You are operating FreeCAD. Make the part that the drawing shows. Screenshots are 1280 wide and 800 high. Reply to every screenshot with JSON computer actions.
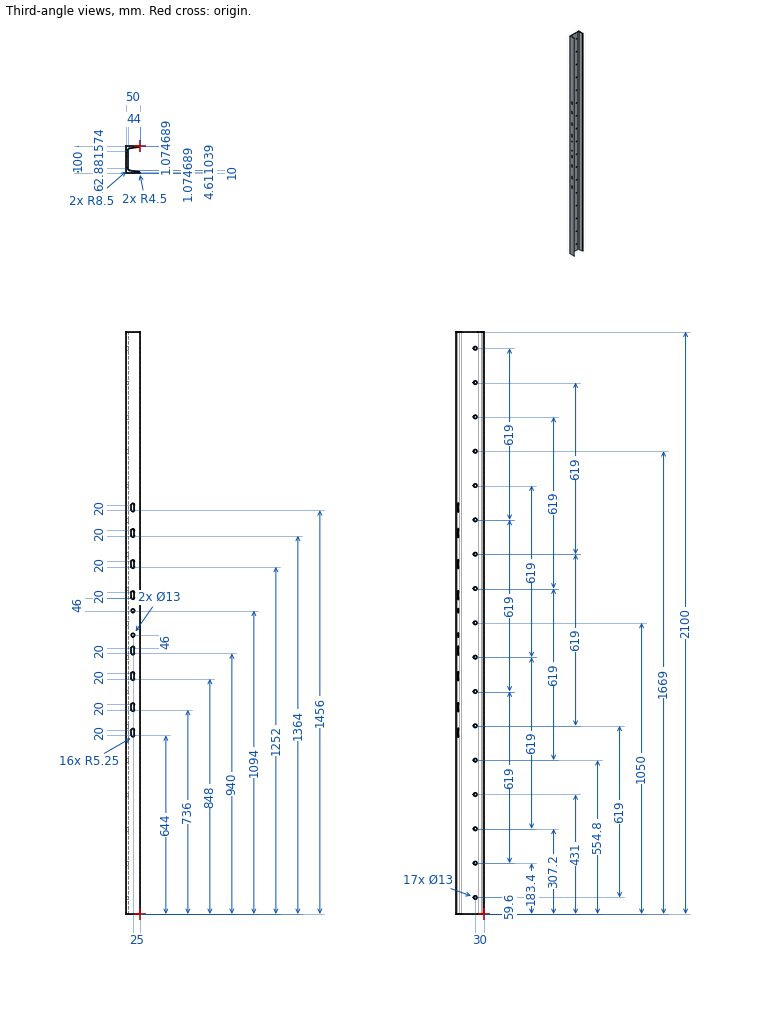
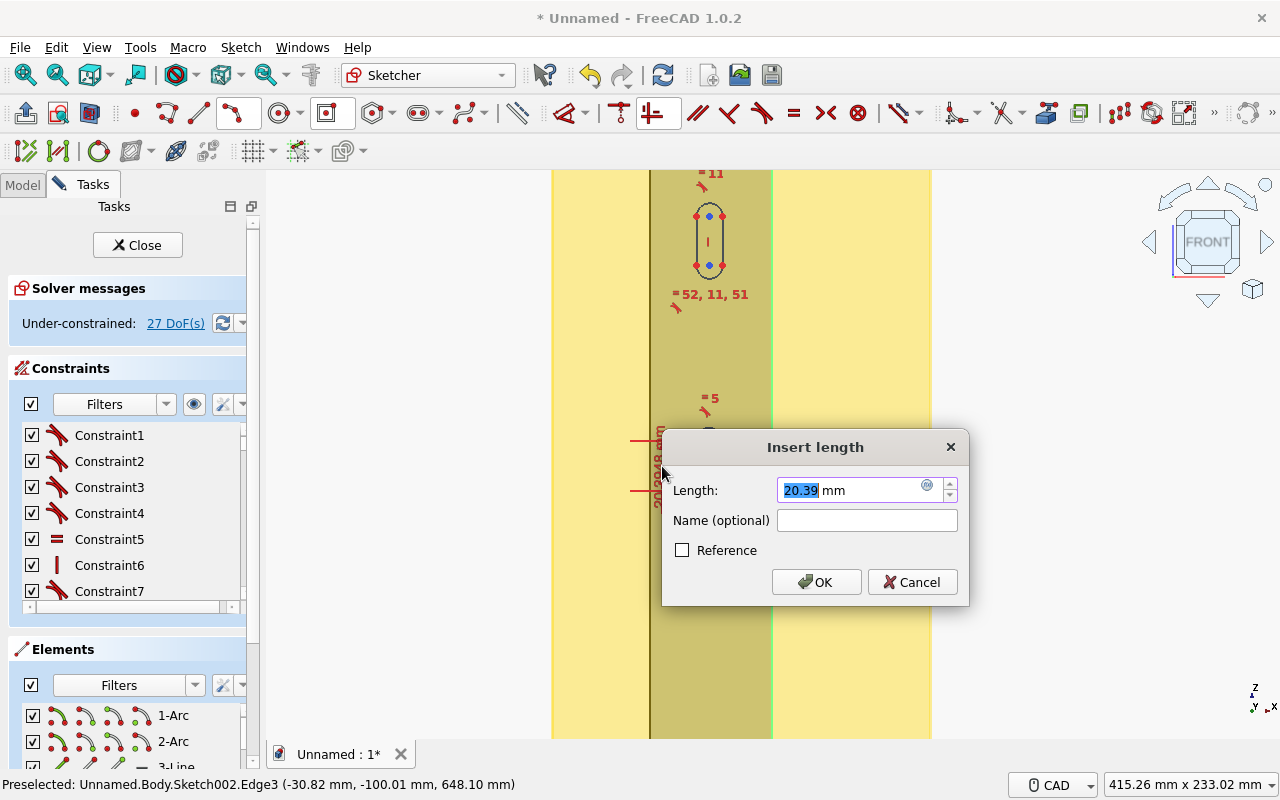
{"action": "type", "text": "20"}
{"action": "key", "text": "Return"}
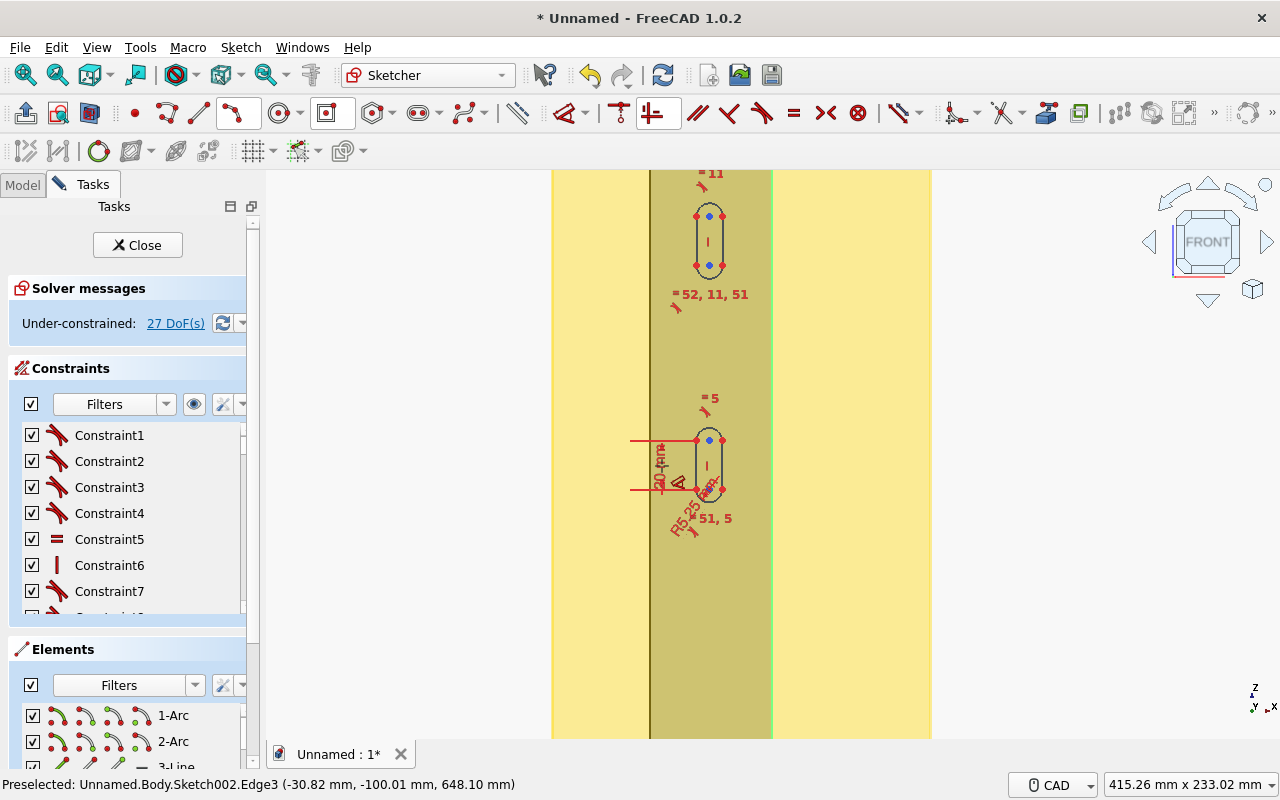
{"action": "left_click", "coordinate": [697, 251]}
{"action": "left_click", "coordinate": [663, 241]}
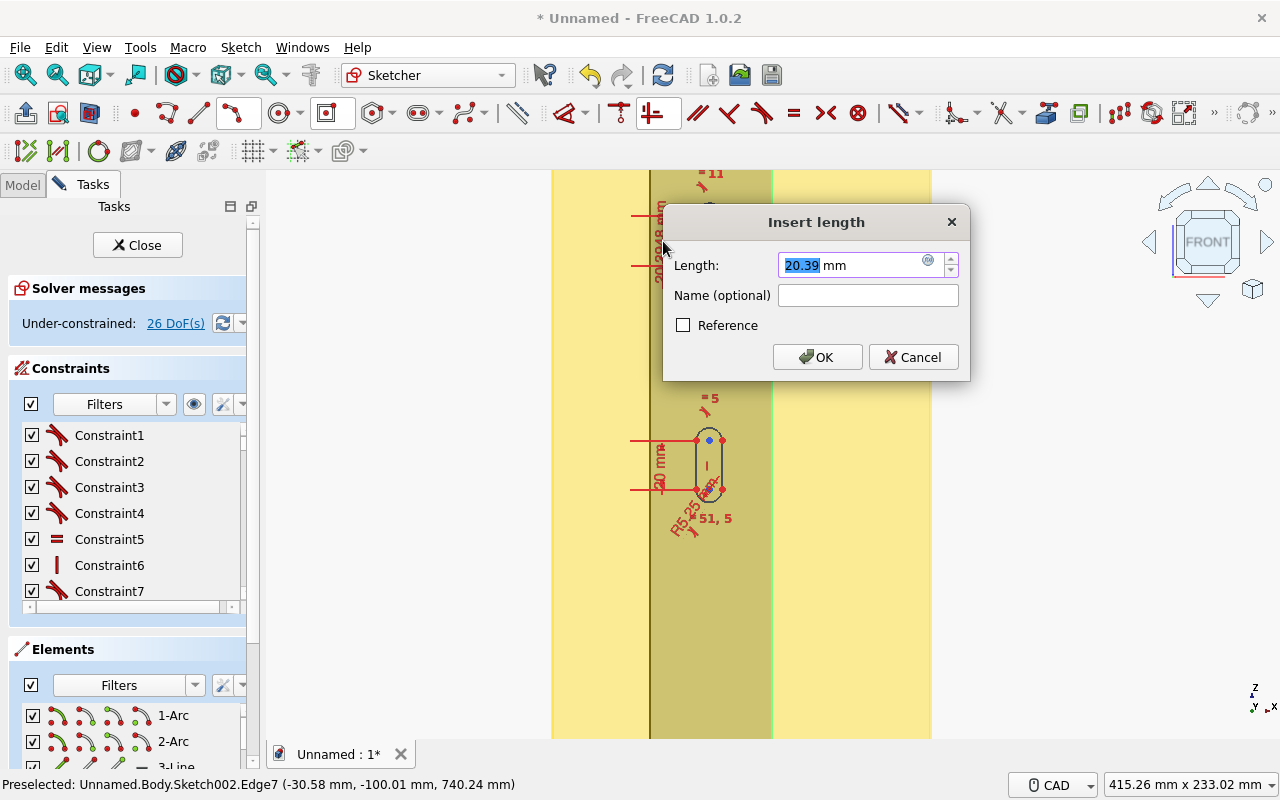
{"action": "type", "text": "20"}
{"action": "key", "text": "Return"}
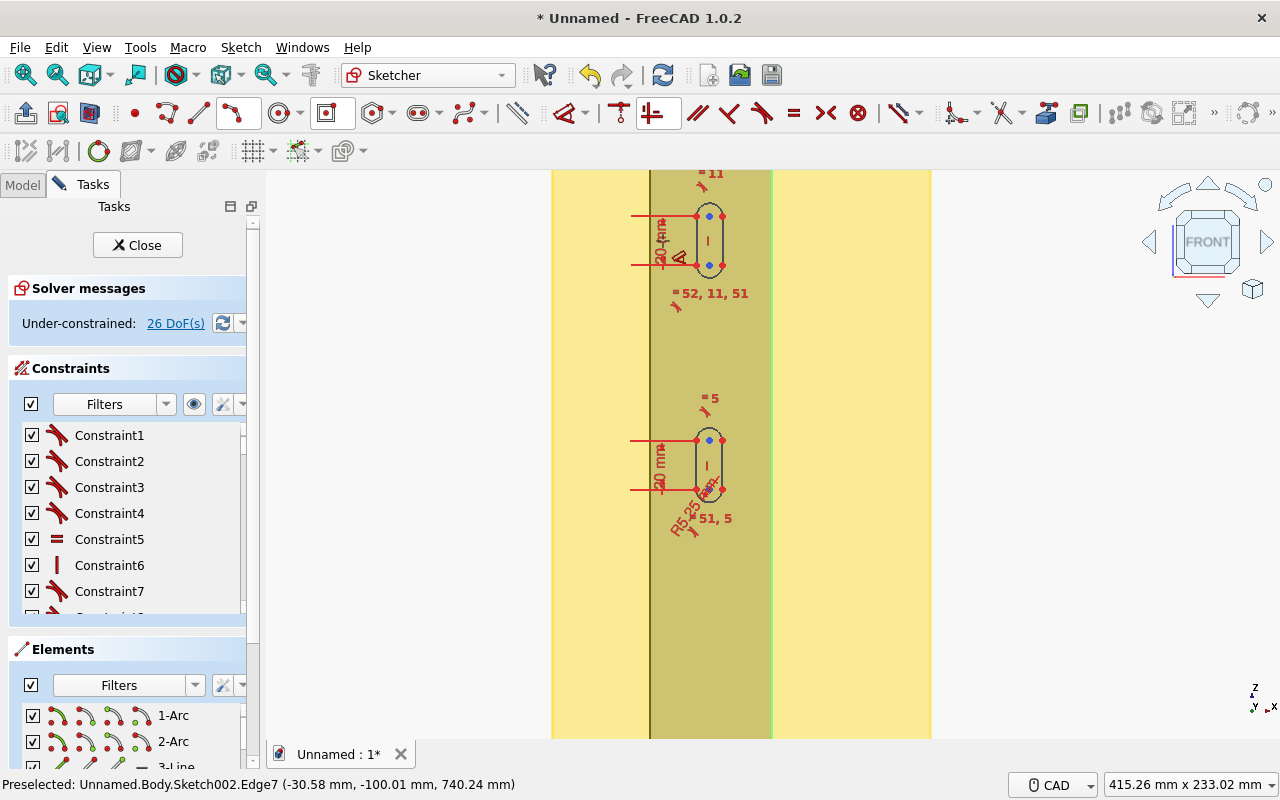
{"action": "scroll", "coordinate": [702, 475], "scroll_direction": "down", "scroll_amount": 12}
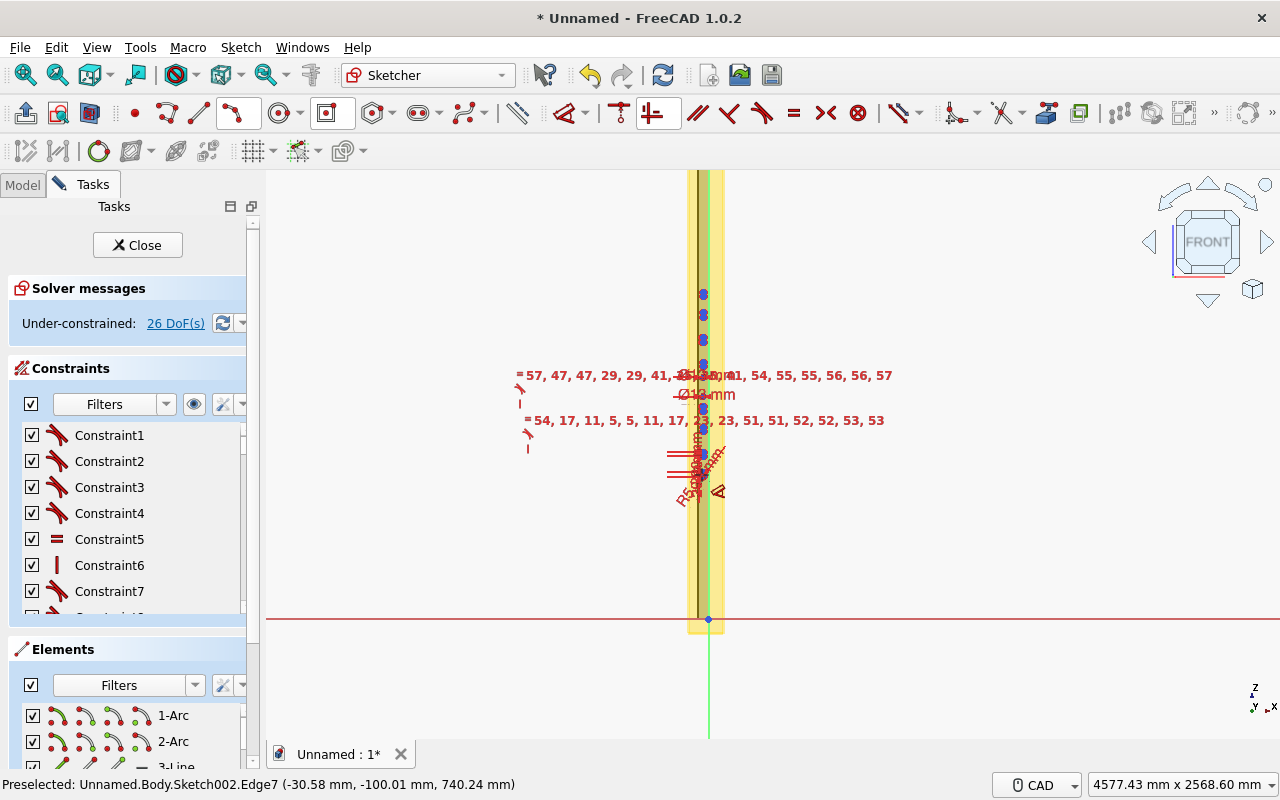
{"action": "scroll", "coordinate": [702, 430], "scroll_direction": "up", "scroll_amount": 12}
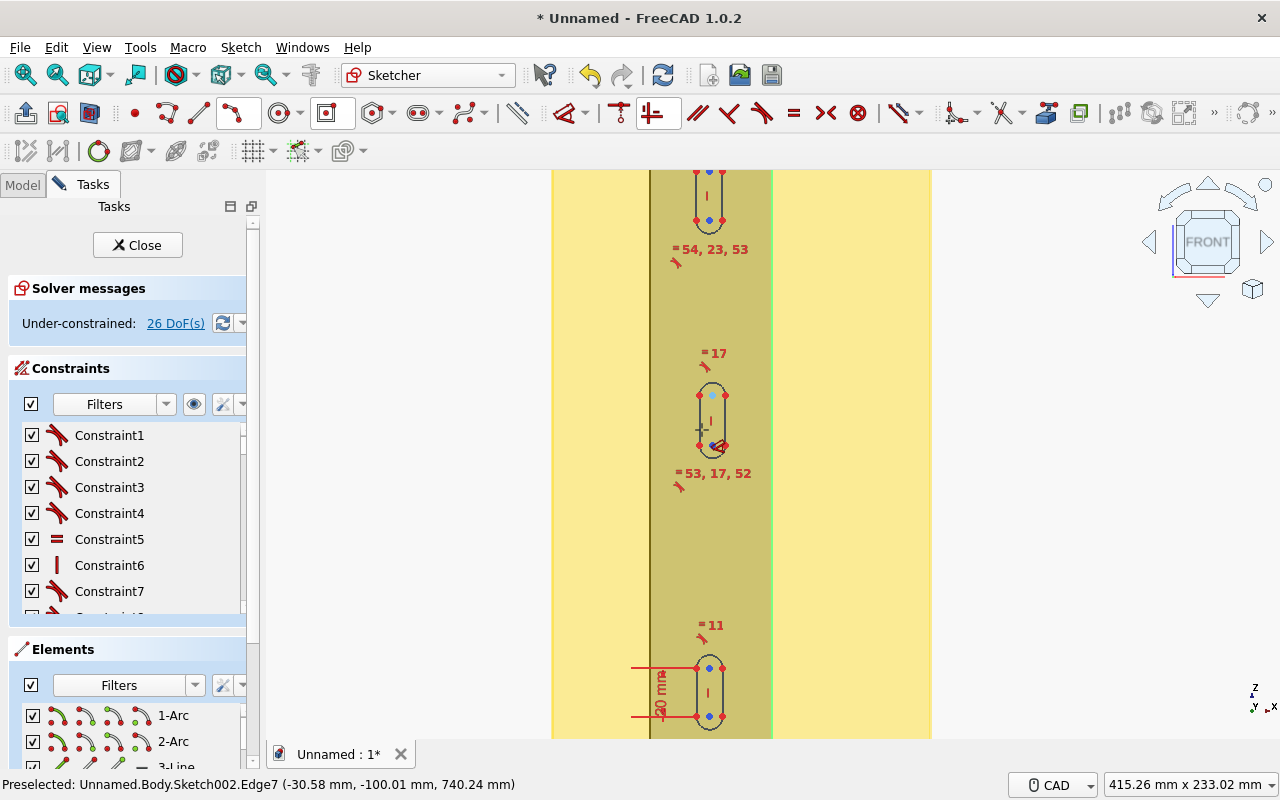
{"action": "left_click", "coordinate": [700, 430]}
{"action": "left_click", "coordinate": [666, 420]}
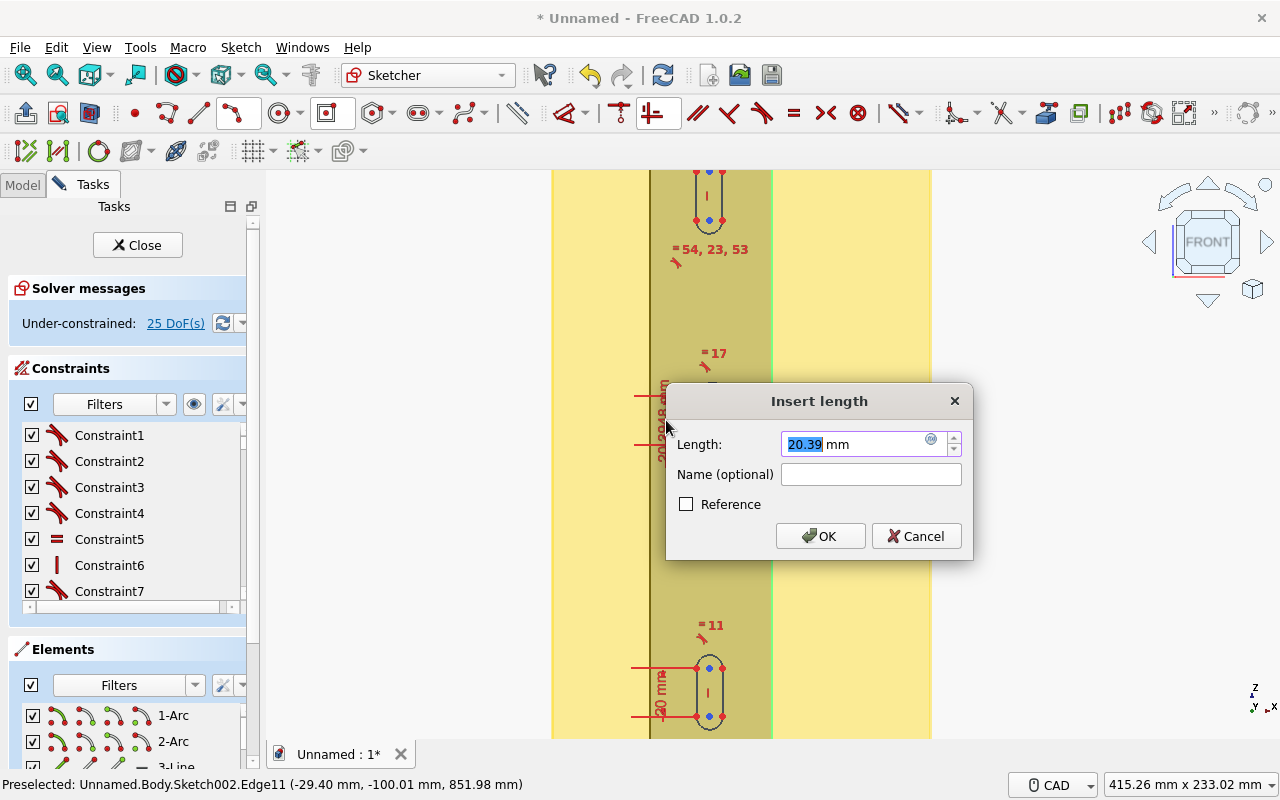
{"action": "type", "text": "20"}
{"action": "key", "text": "Return"}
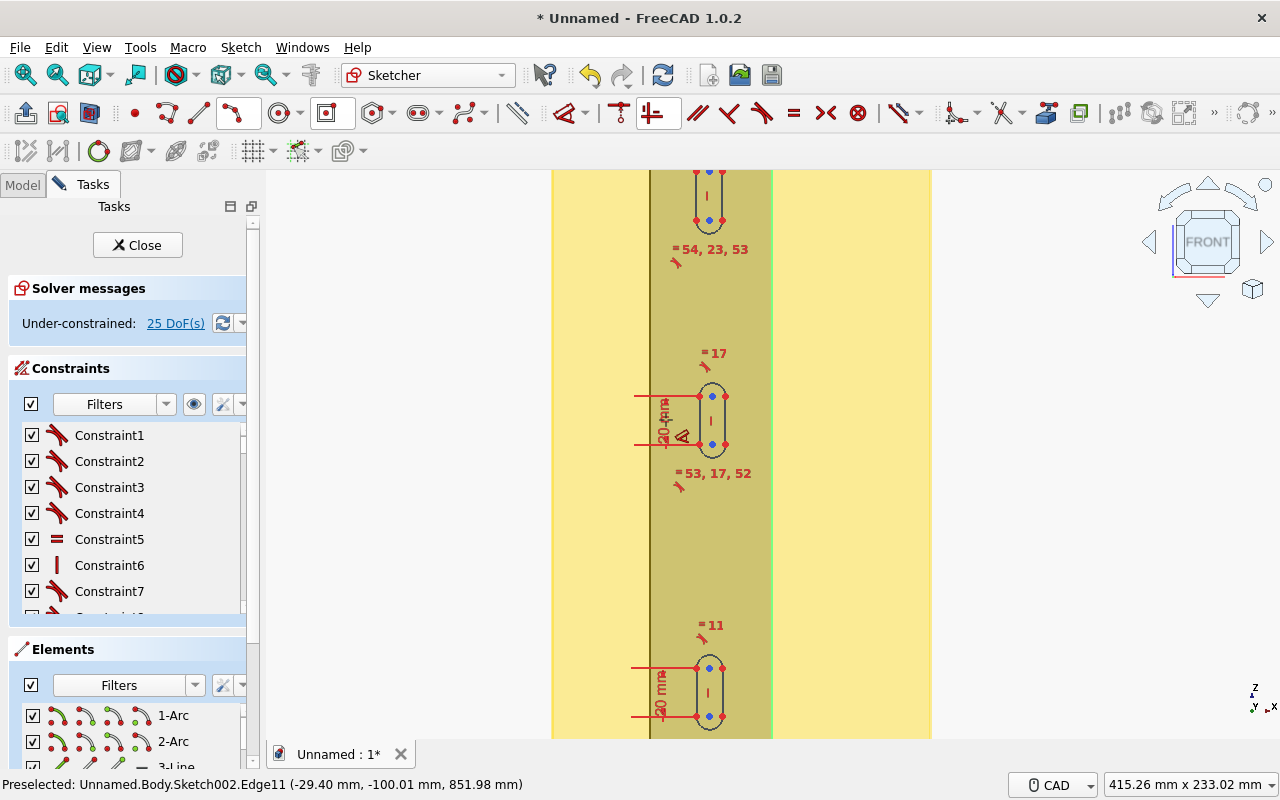
{"action": "left_click", "coordinate": [696, 206]}
{"action": "left_click", "coordinate": [662, 209]}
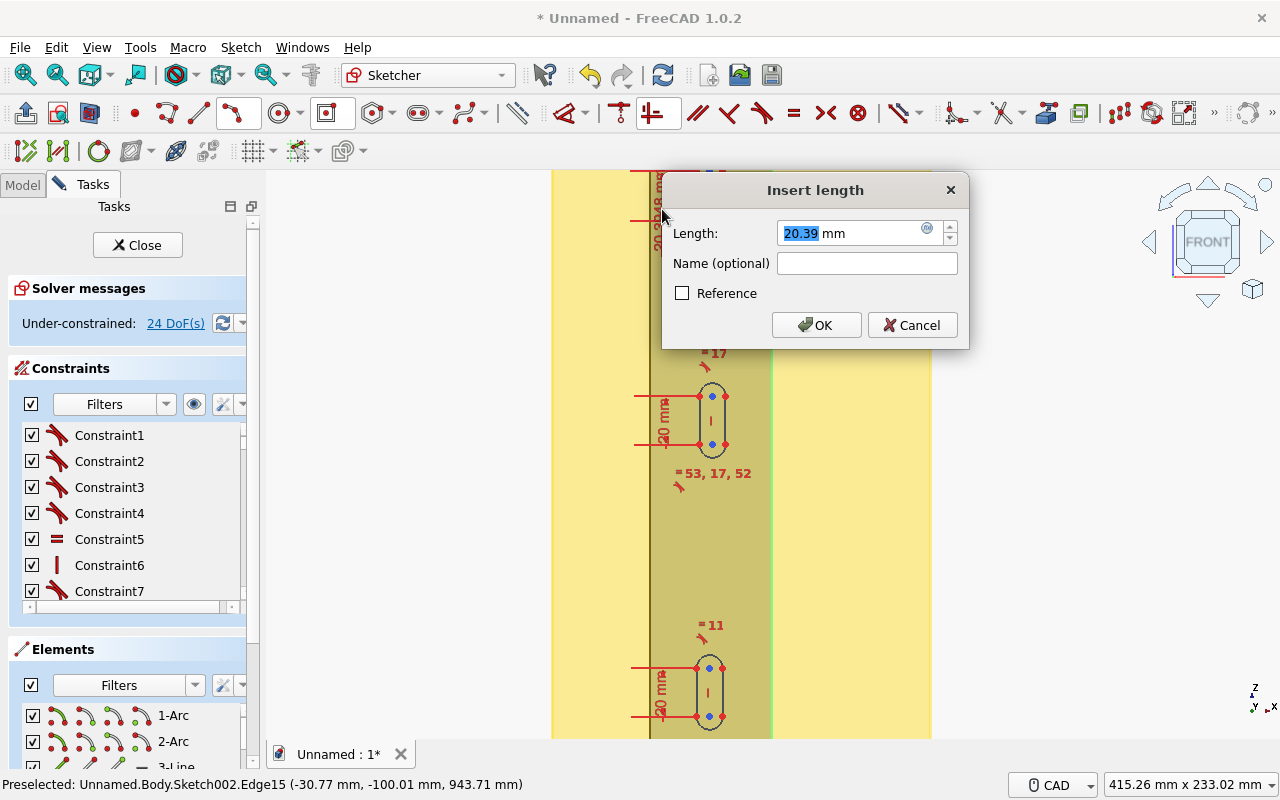
{"action": "type", "text": "20"}
{"action": "key", "text": "Return"}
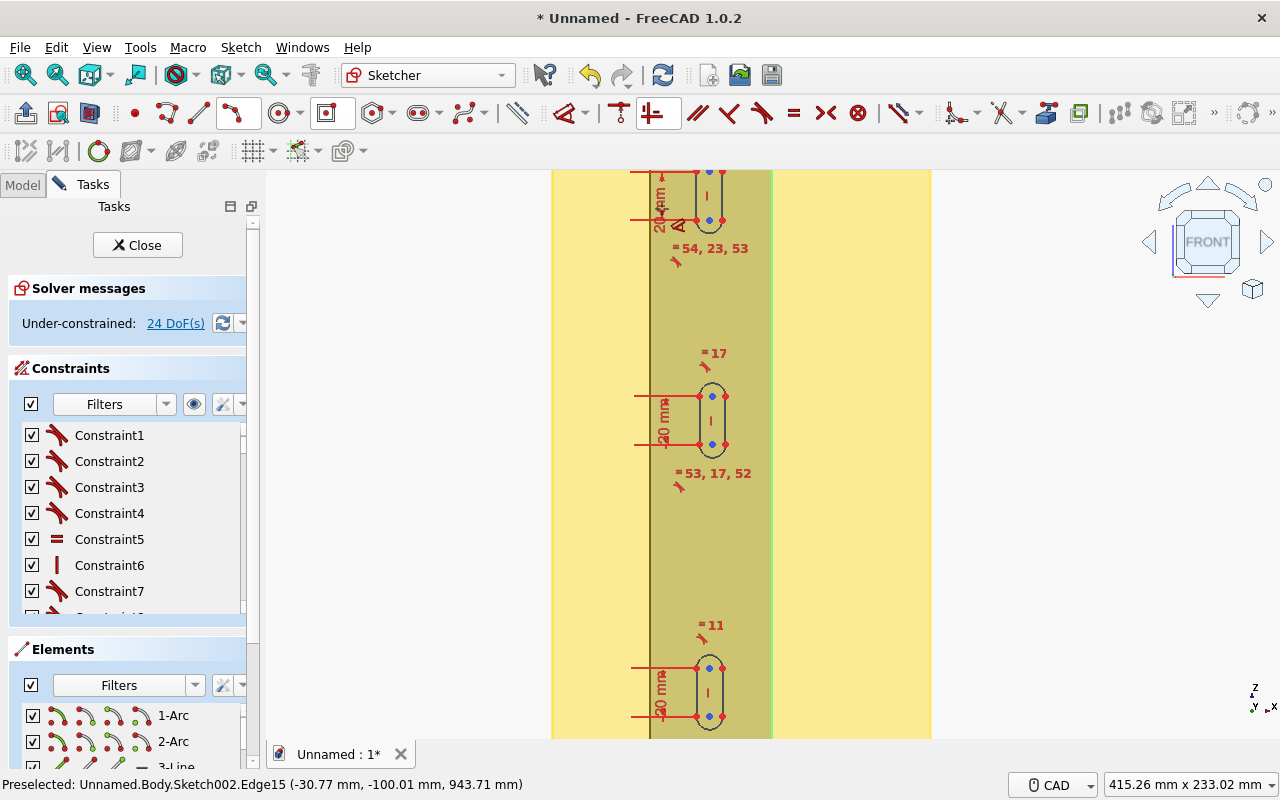
{"action": "scroll", "coordinate": [702, 430], "scroll_direction": "down", "scroll_amount": 12}